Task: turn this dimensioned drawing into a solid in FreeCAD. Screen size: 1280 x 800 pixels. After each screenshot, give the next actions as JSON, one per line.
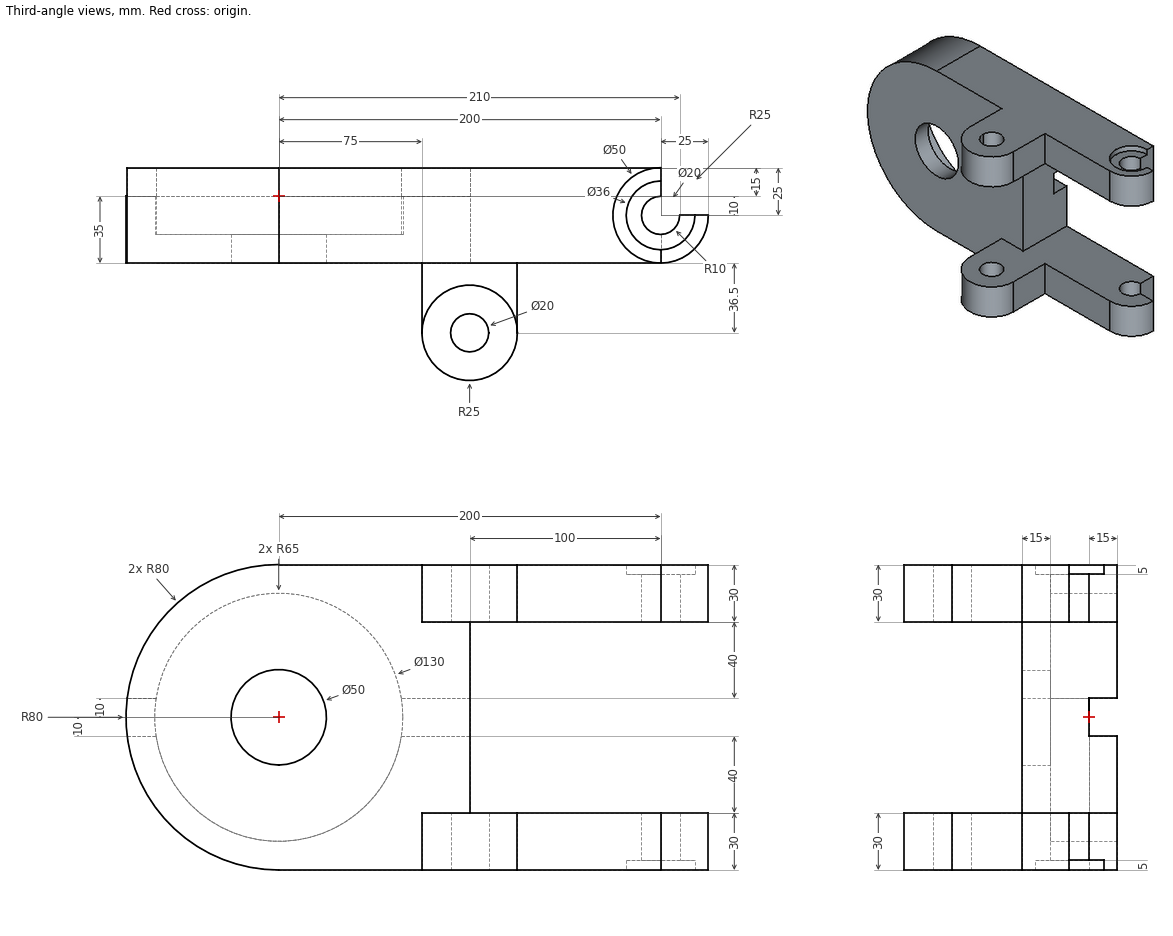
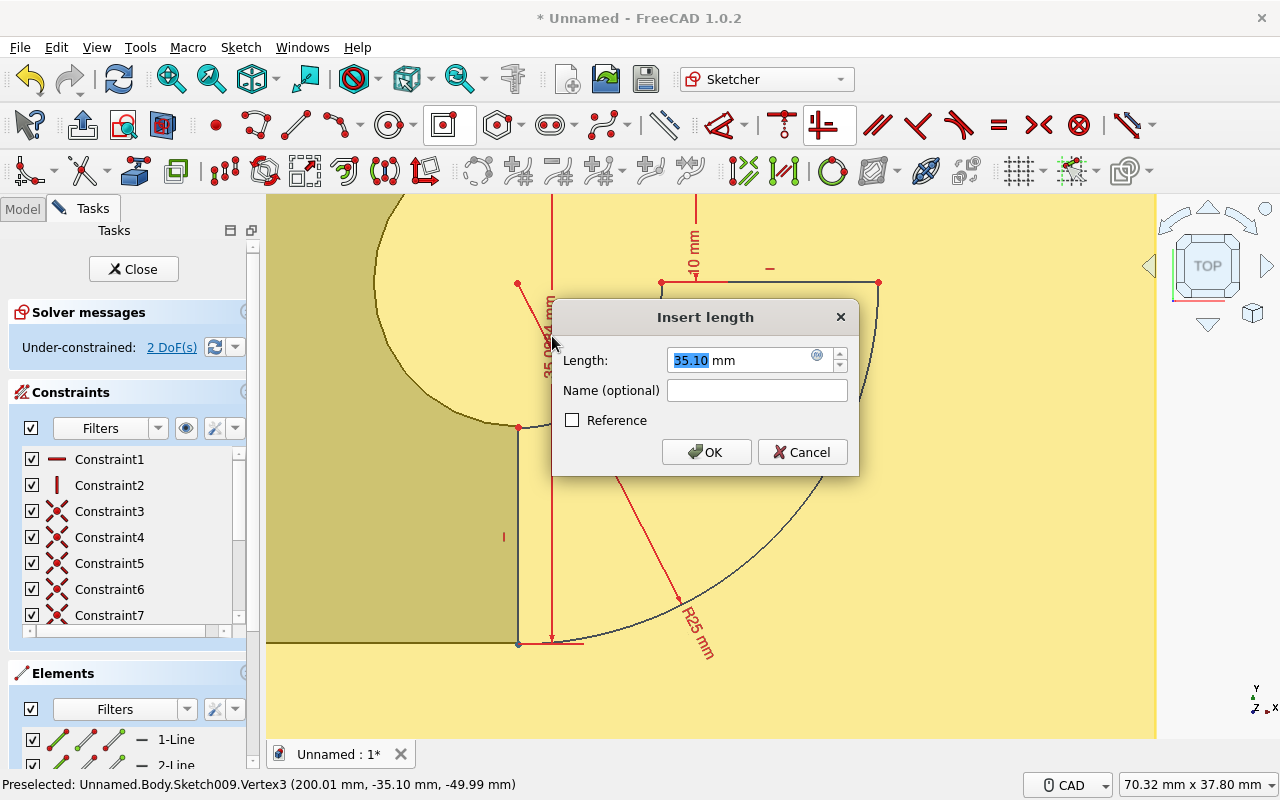
{"action": "type", "text": "35"}
{"action": "key", "text": "Return"}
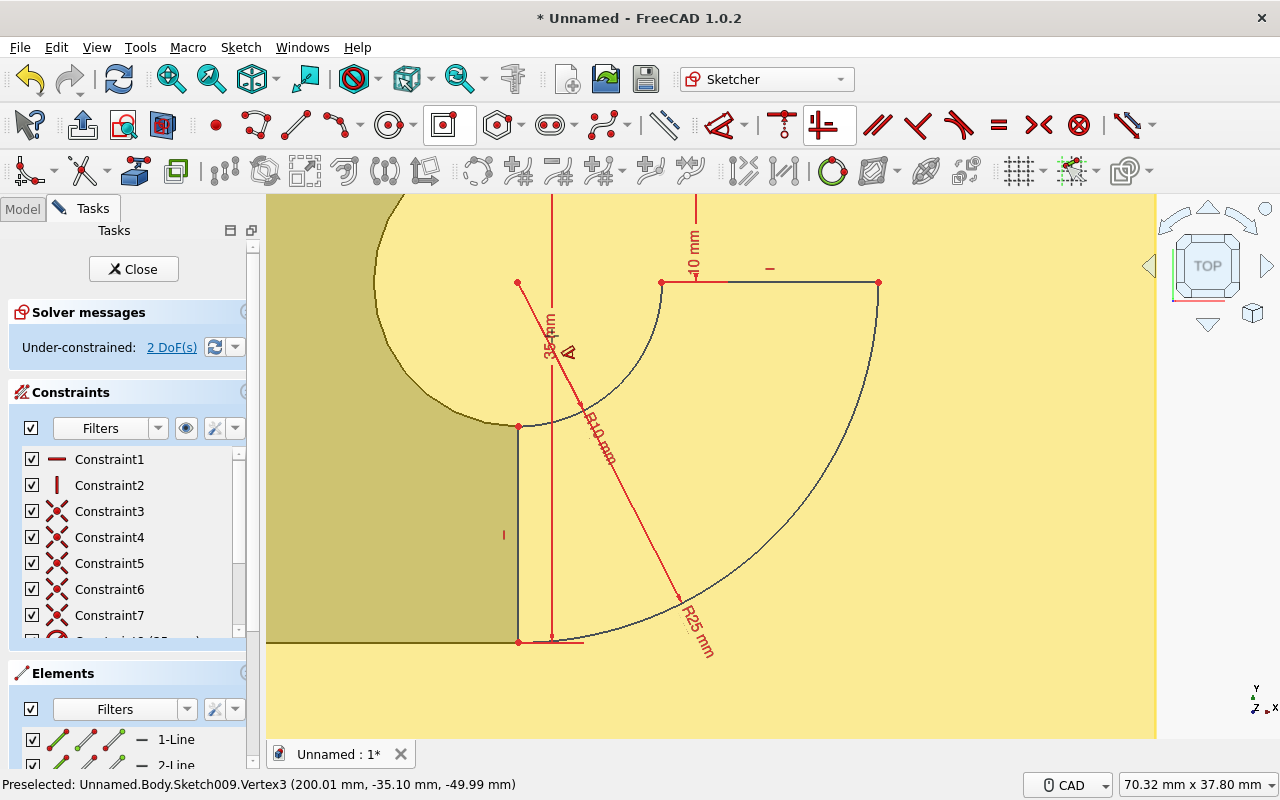
{"action": "left_click", "coordinate": [662, 282]}
{"action": "left_click", "coordinate": [478, 316]}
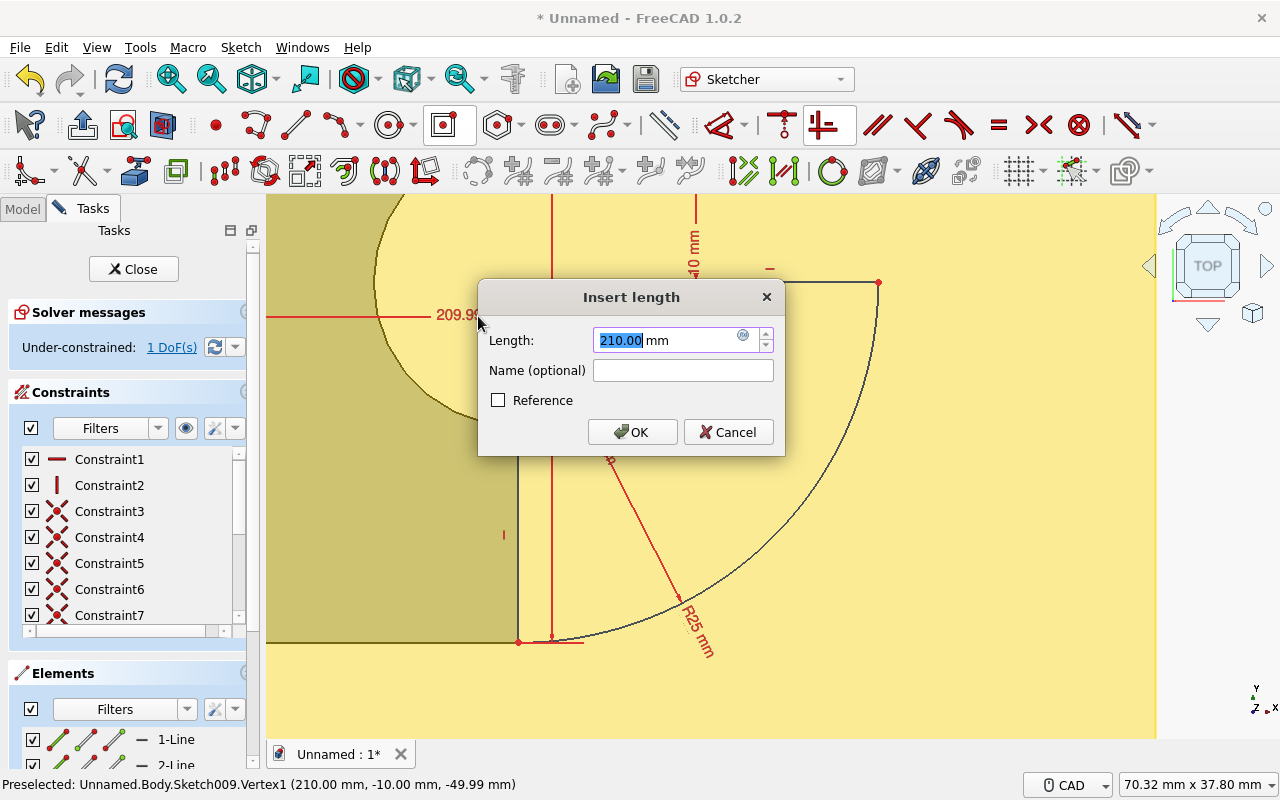
{"action": "type", "text": "210"}
{"action": "key", "text": "Return"}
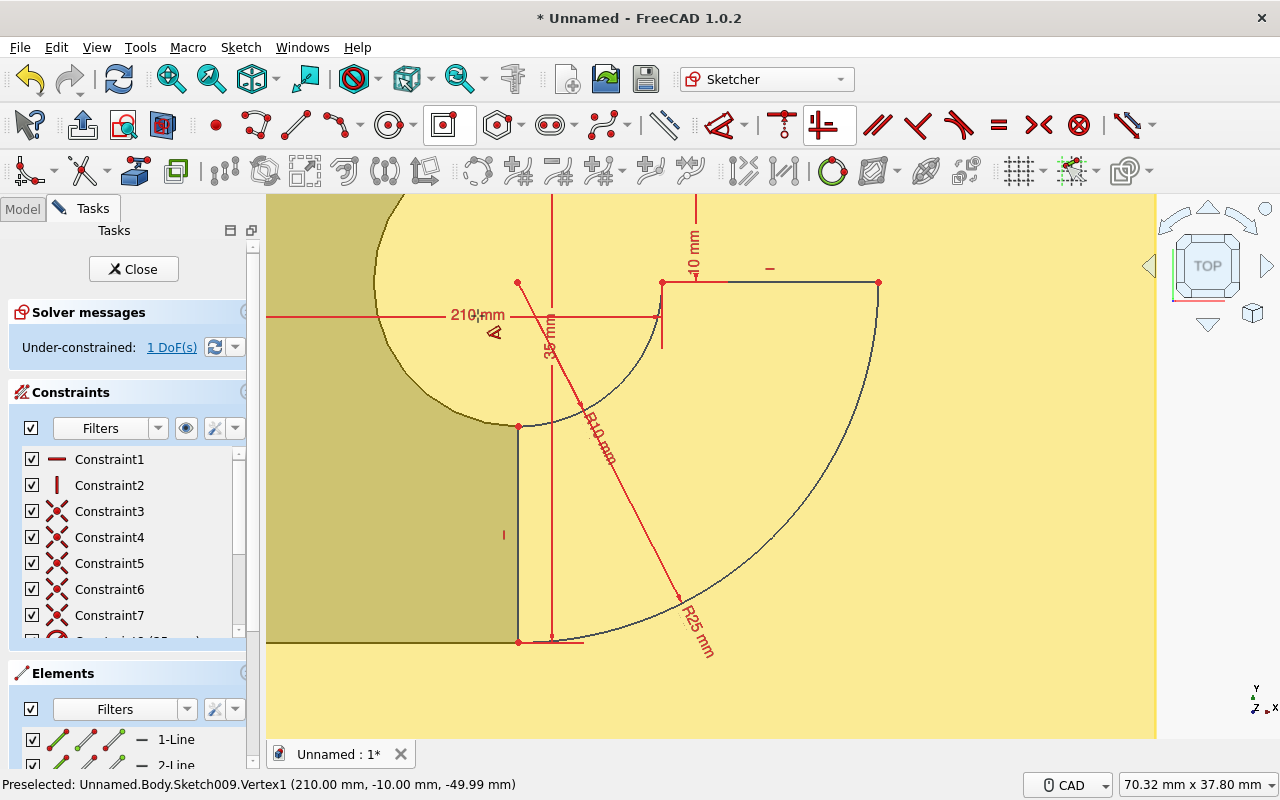
{"action": "left_click", "coordinate": [518, 643]}
{"action": "left_click", "coordinate": [406, 677]}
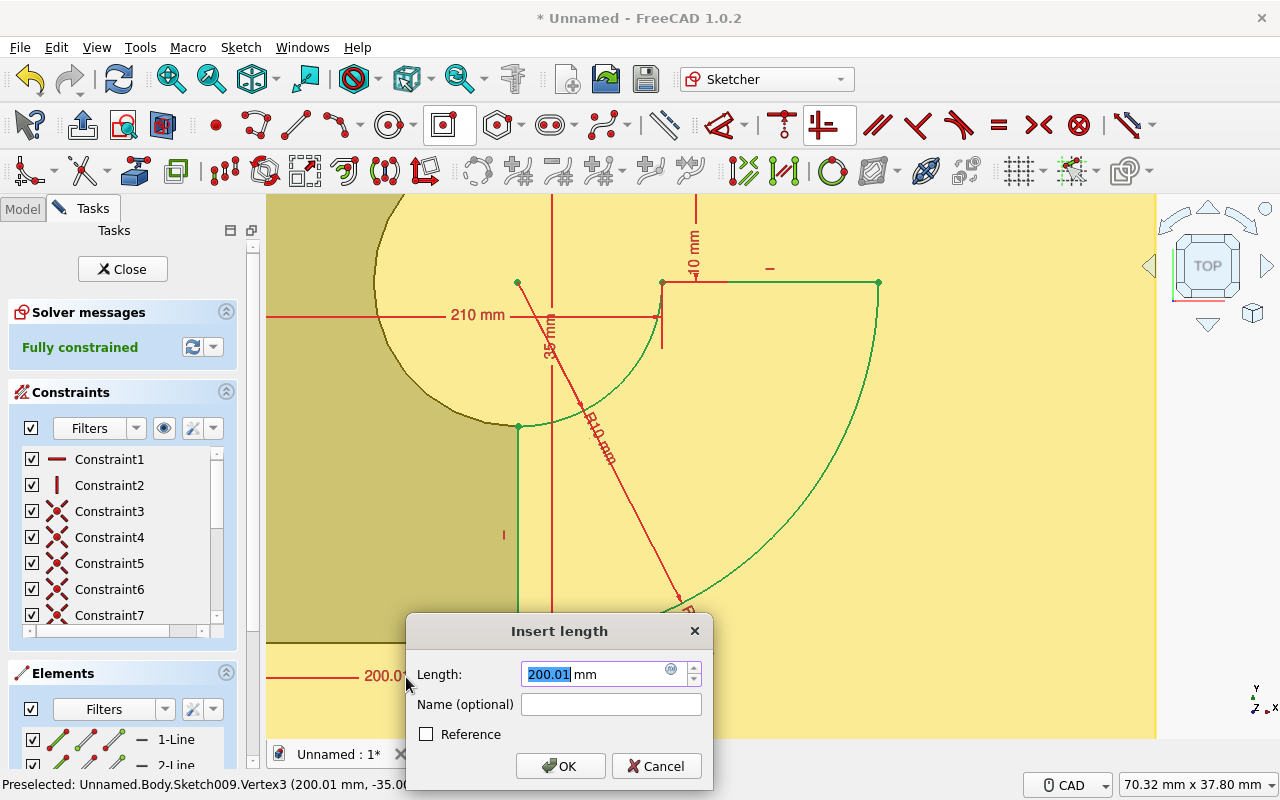
{"action": "type", "text": "200"}
{"action": "key", "text": "Return"}
{"action": "key", "text": "Escape"}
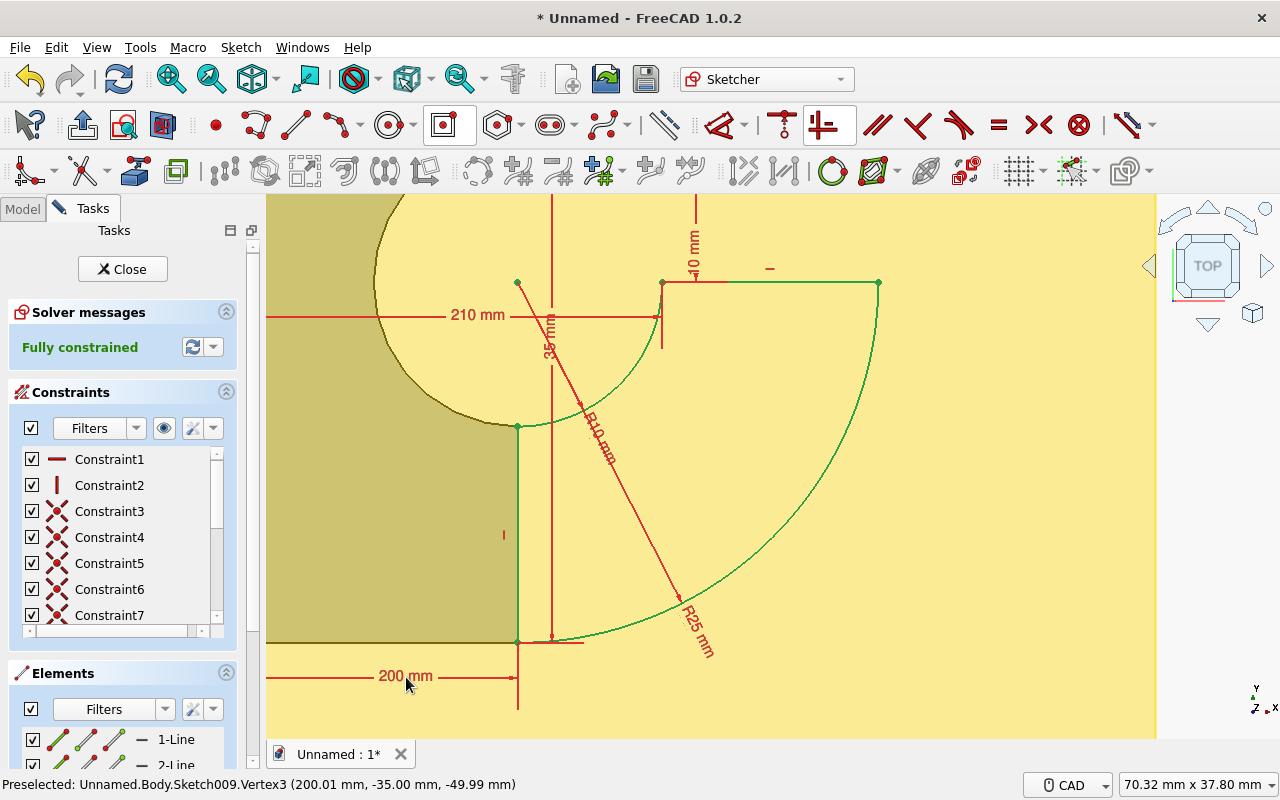
{"action": "left_click", "coordinate": [123, 269]}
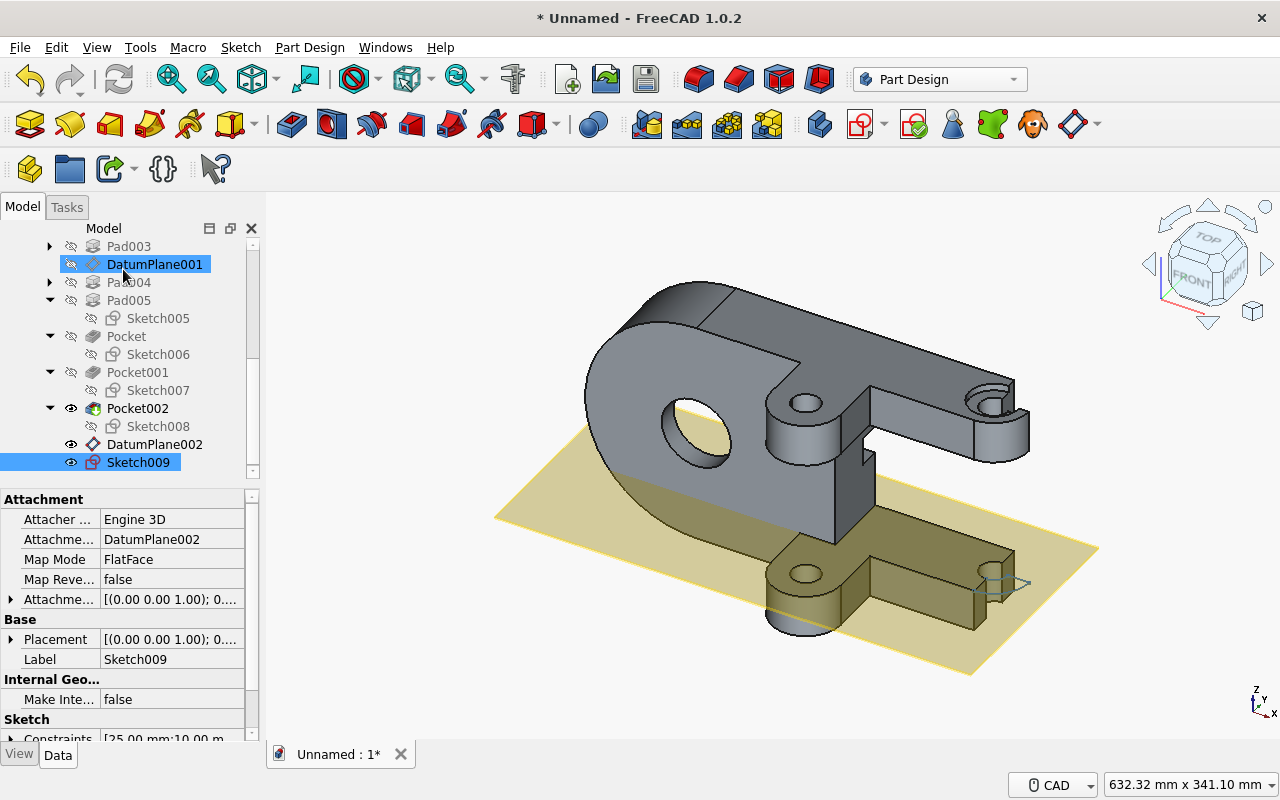
{"action": "left_click", "coordinate": [30, 124]}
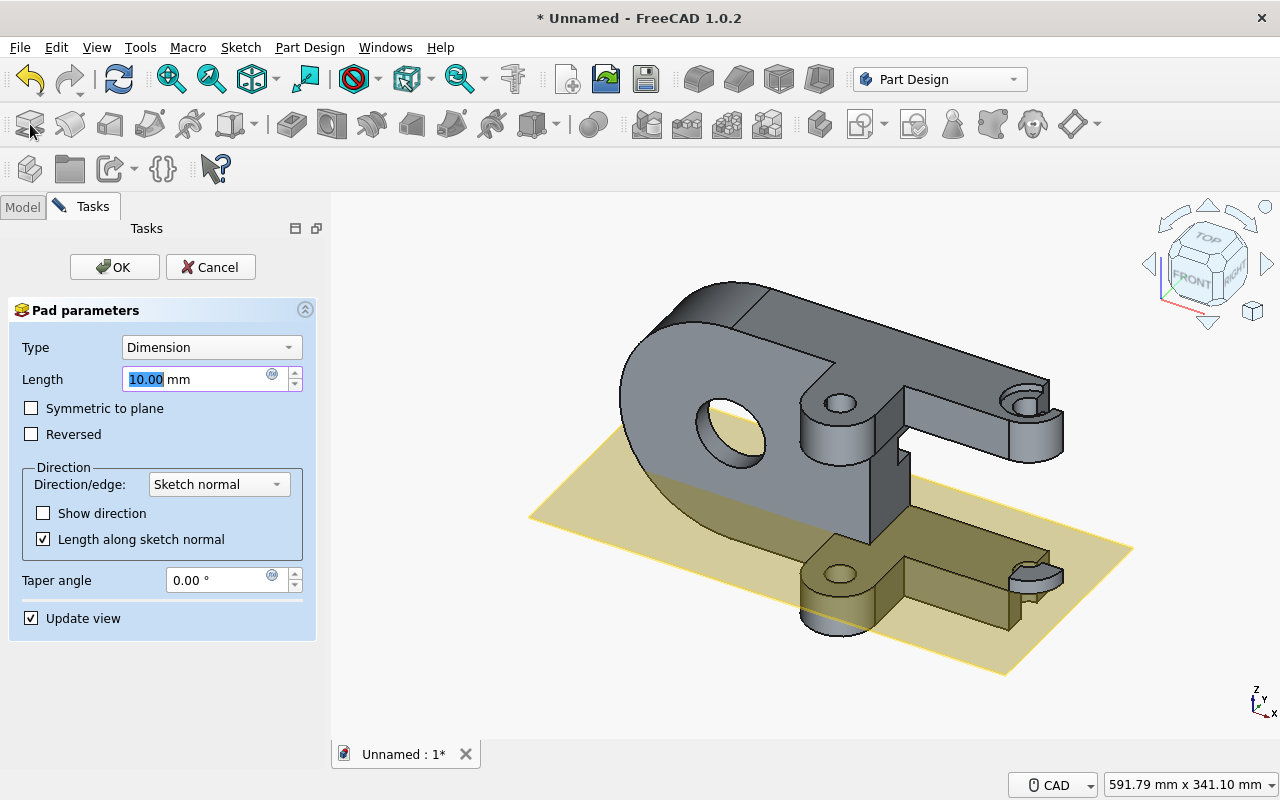
{"action": "type", "text": "30"}
{"action": "key", "text": "Tab"}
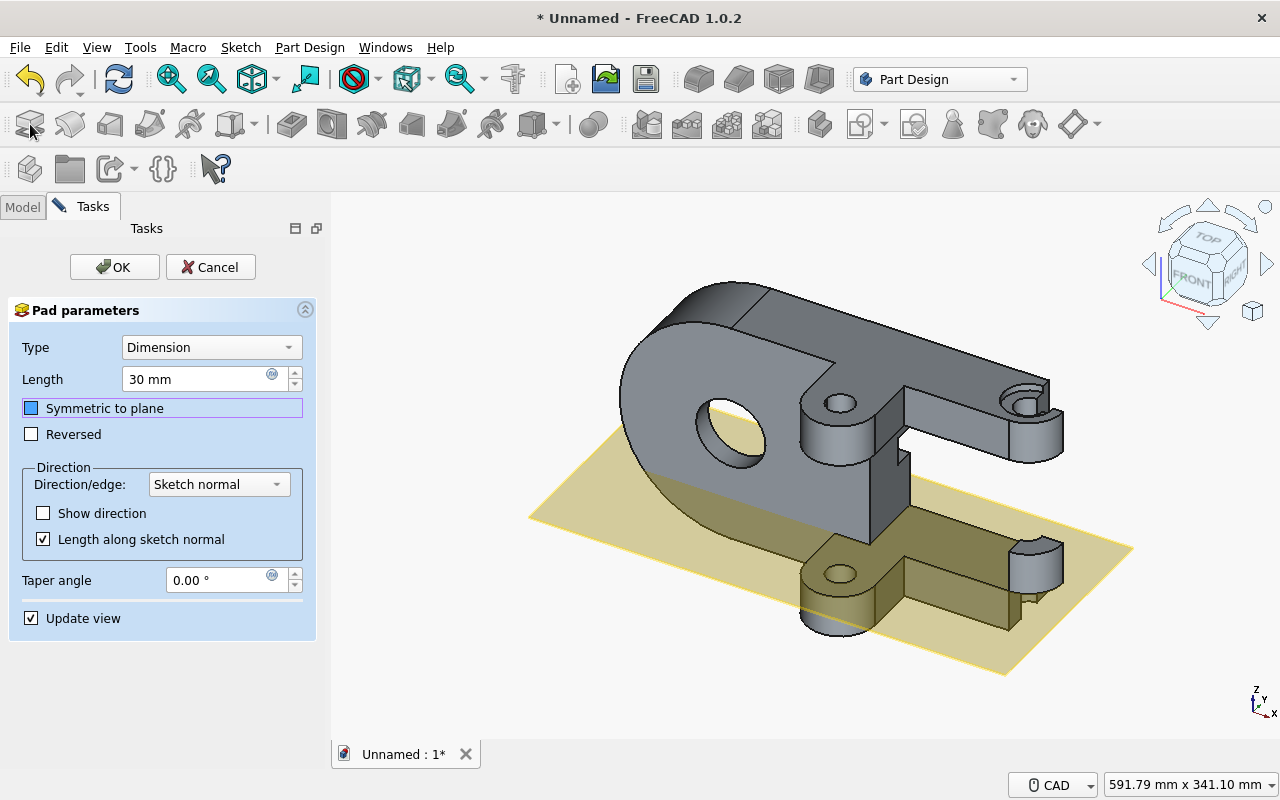
{"action": "left_click", "coordinate": [30, 434]}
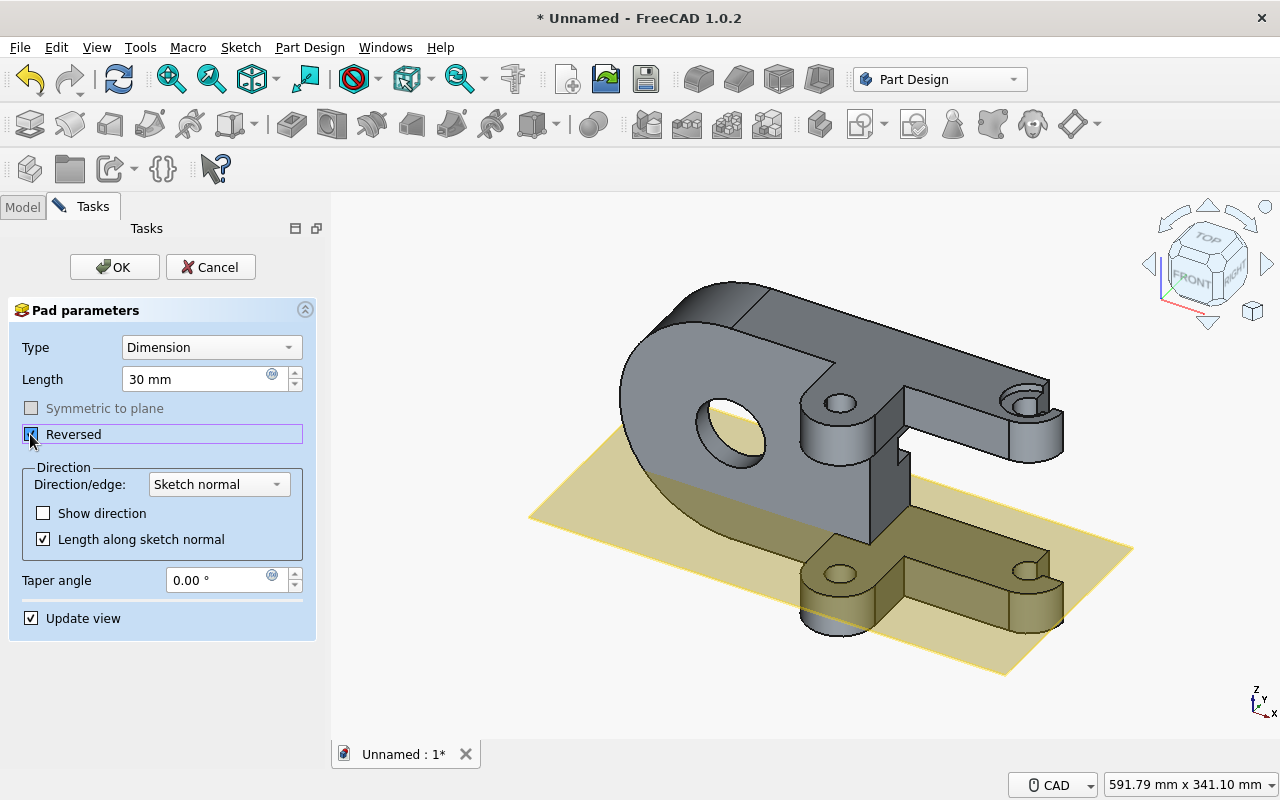
{"action": "left_click", "coordinate": [115, 267]}